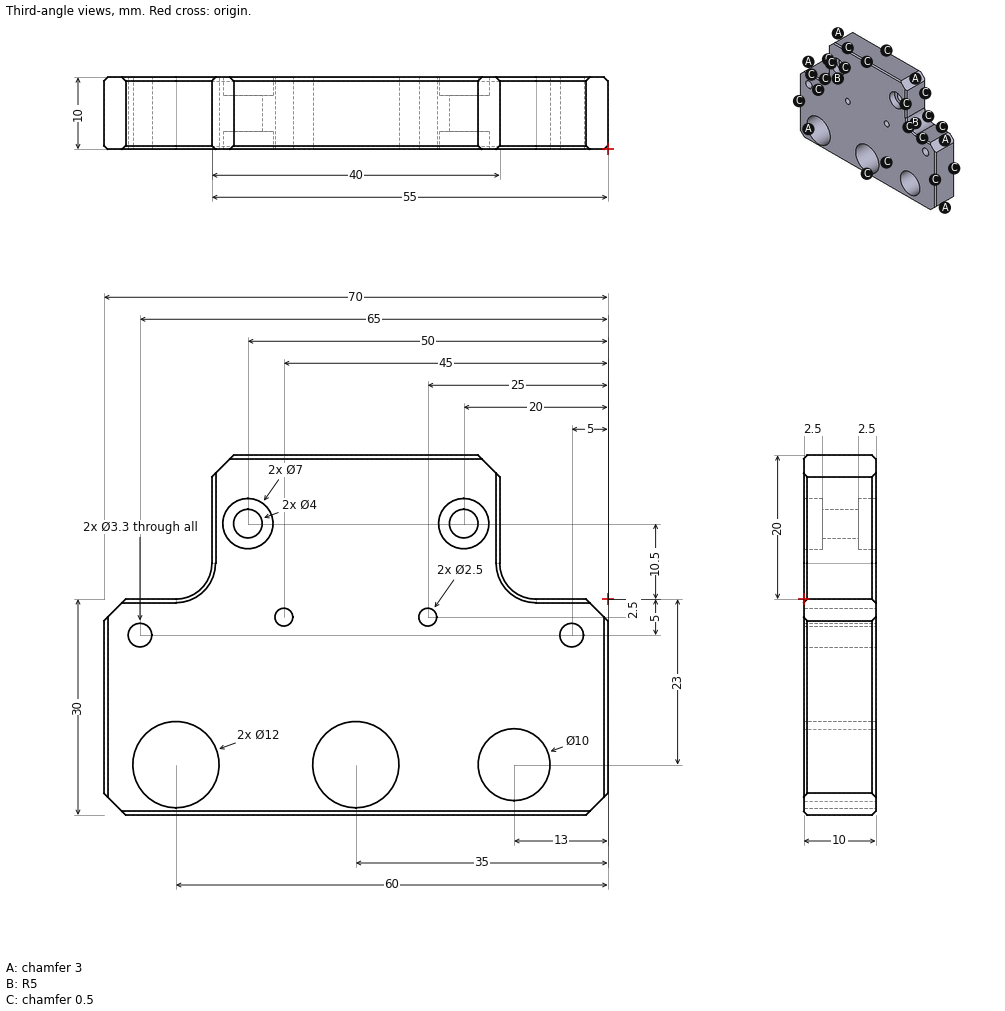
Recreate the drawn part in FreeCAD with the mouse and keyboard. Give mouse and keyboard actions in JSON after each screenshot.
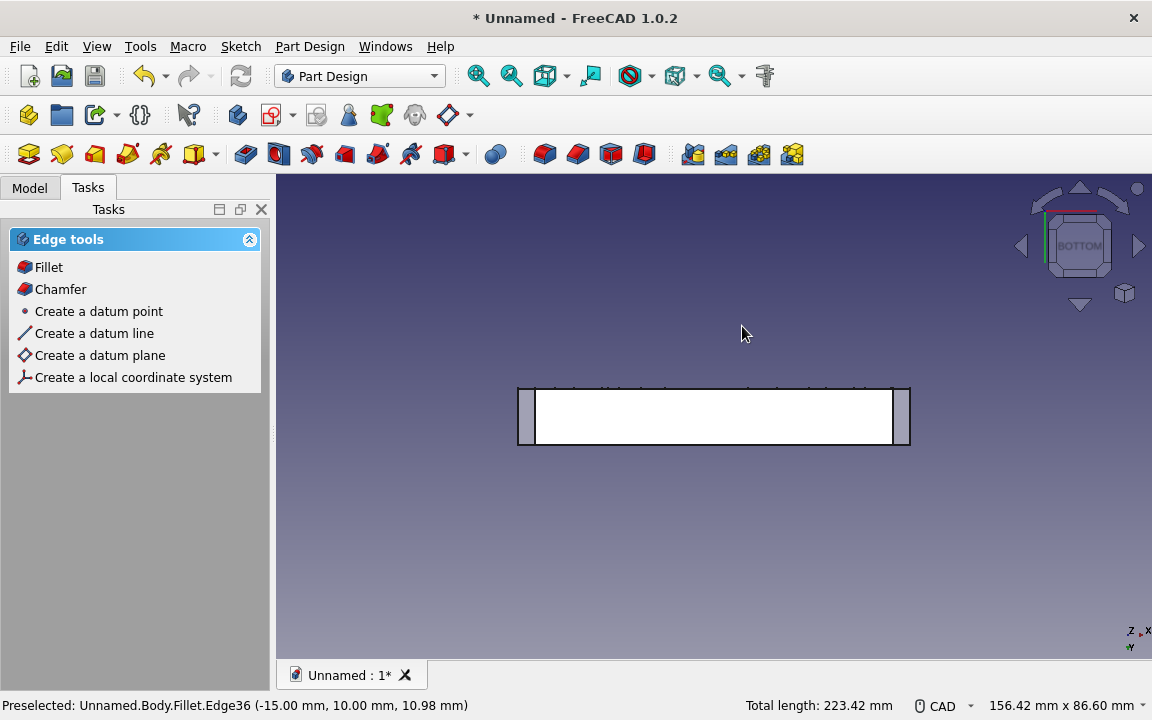
{"action": "left_click", "coordinate": [479, 76]}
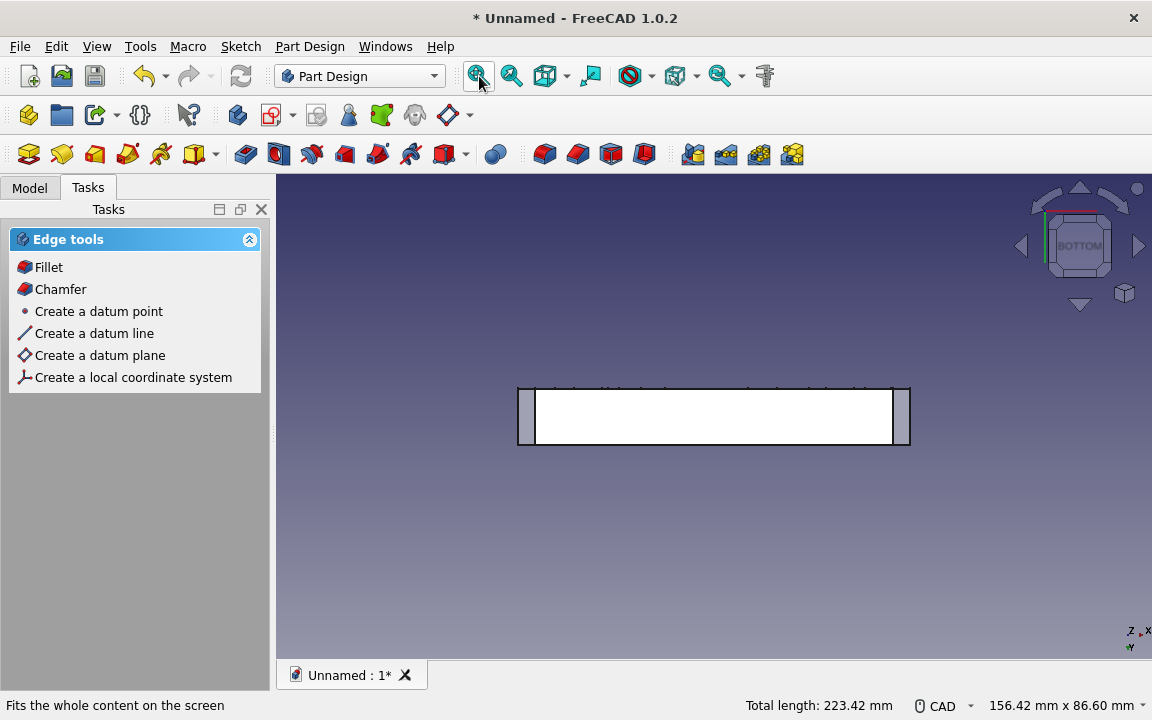
{"action": "left_click", "coordinate": [714, 387], "text": "ctrl"}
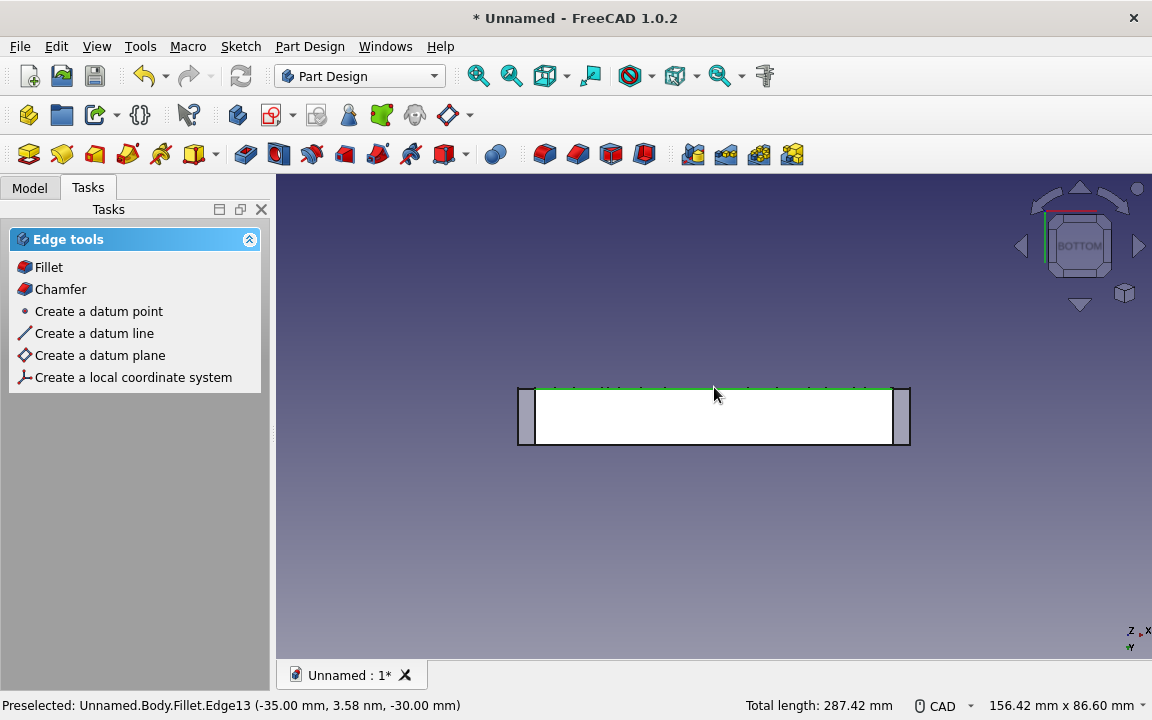
{"action": "key", "text": "4"}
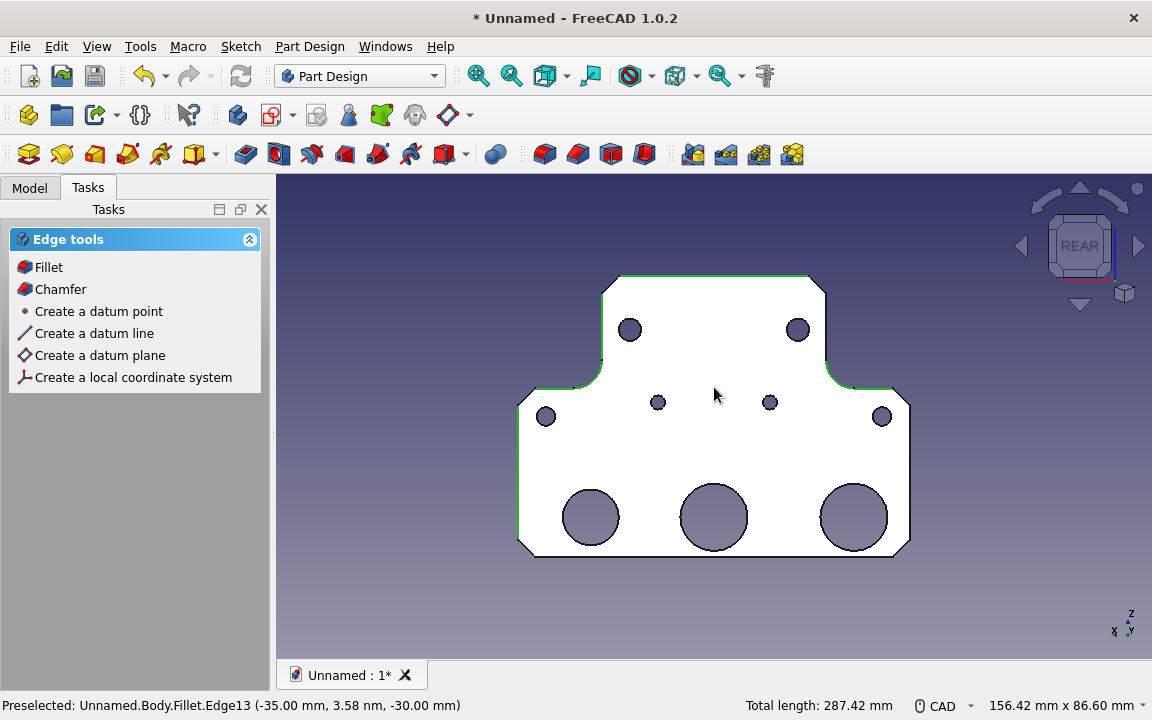
{"action": "left_click", "coordinate": [714, 556], "text": "ctrl"}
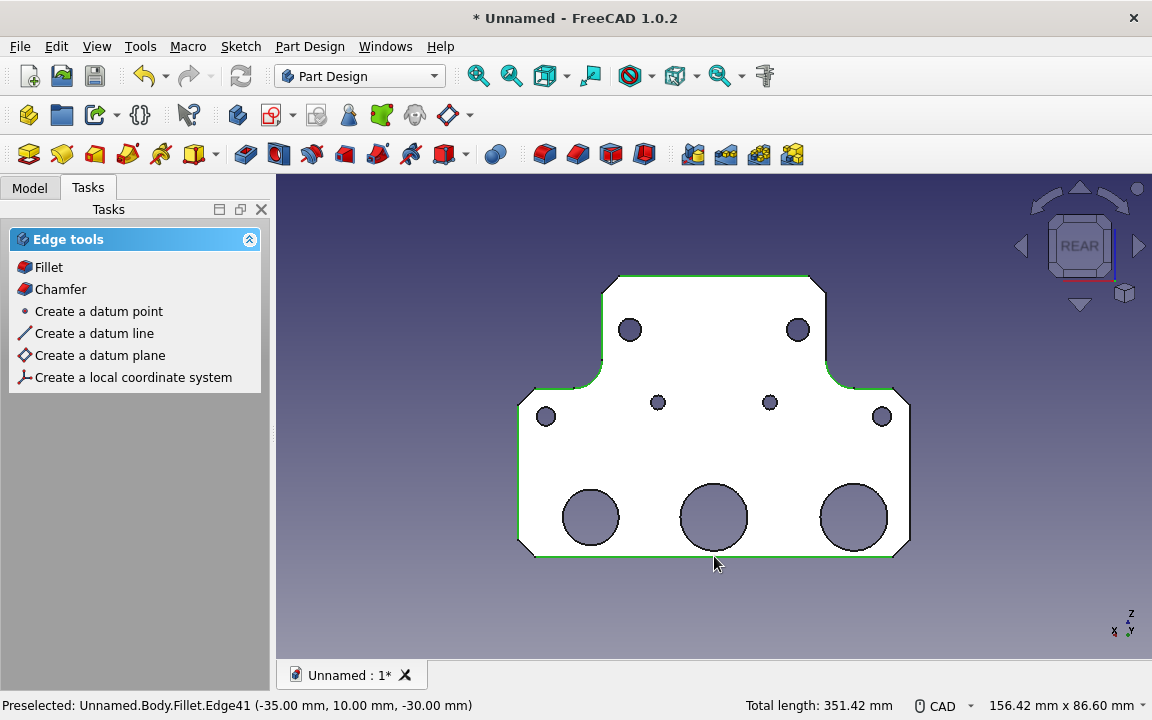
{"action": "left_click", "coordinate": [910, 472], "text": "ctrl"}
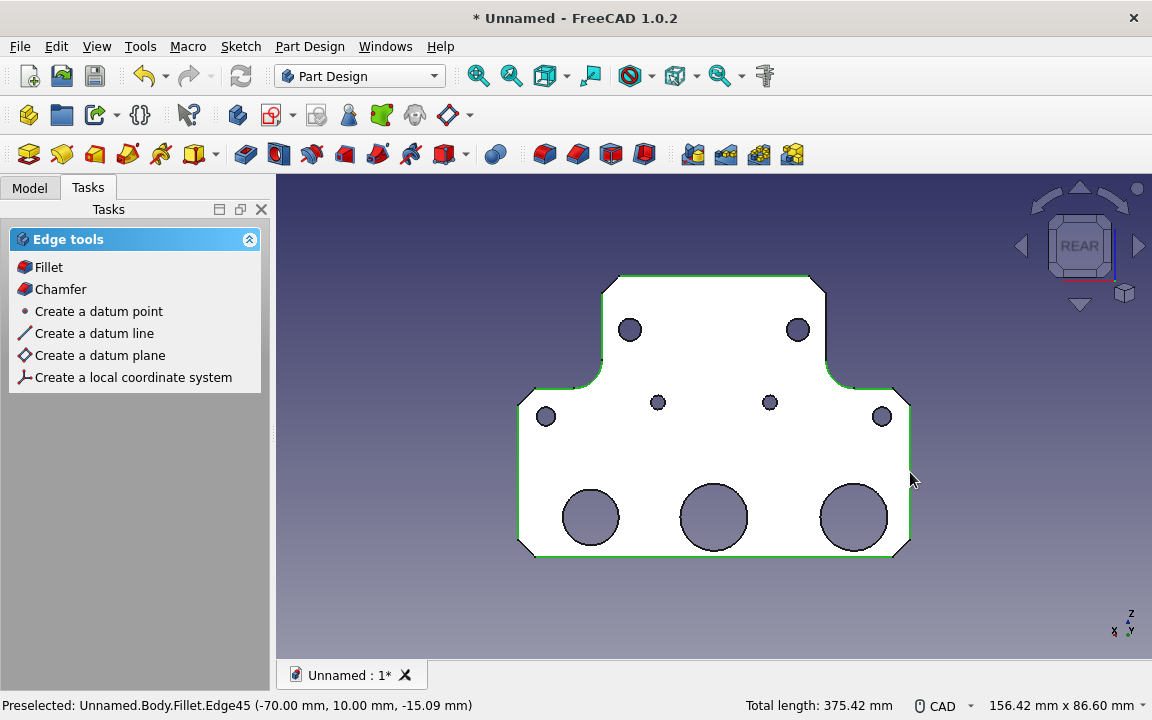
{"action": "left_click", "coordinate": [826, 326], "text": "ctrl"}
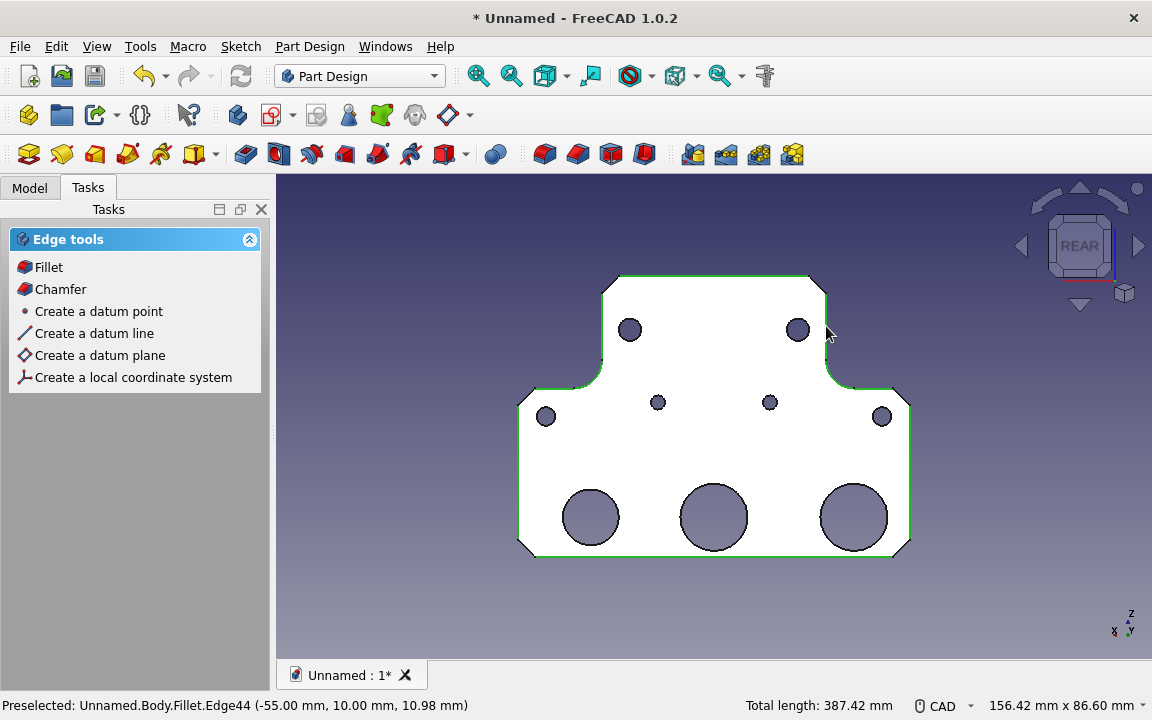
{"action": "key", "text": "6"}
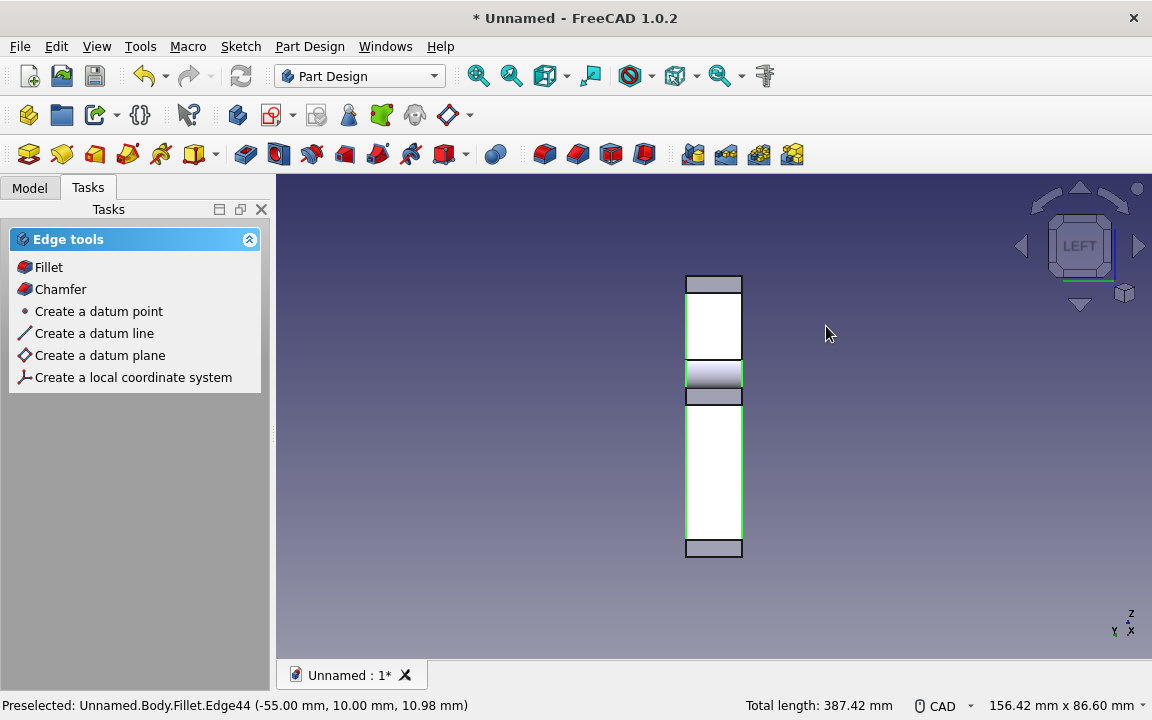
{"action": "left_click", "coordinate": [742, 326], "text": "ctrl"}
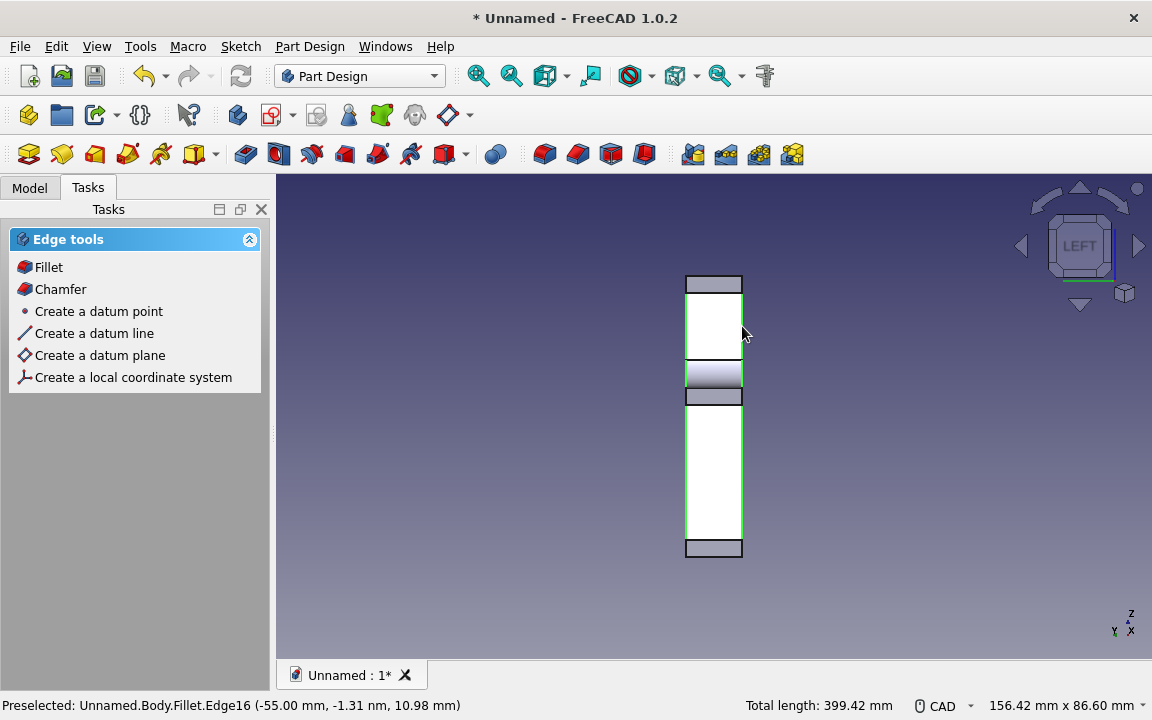
{"action": "left_click", "coordinate": [578, 154]}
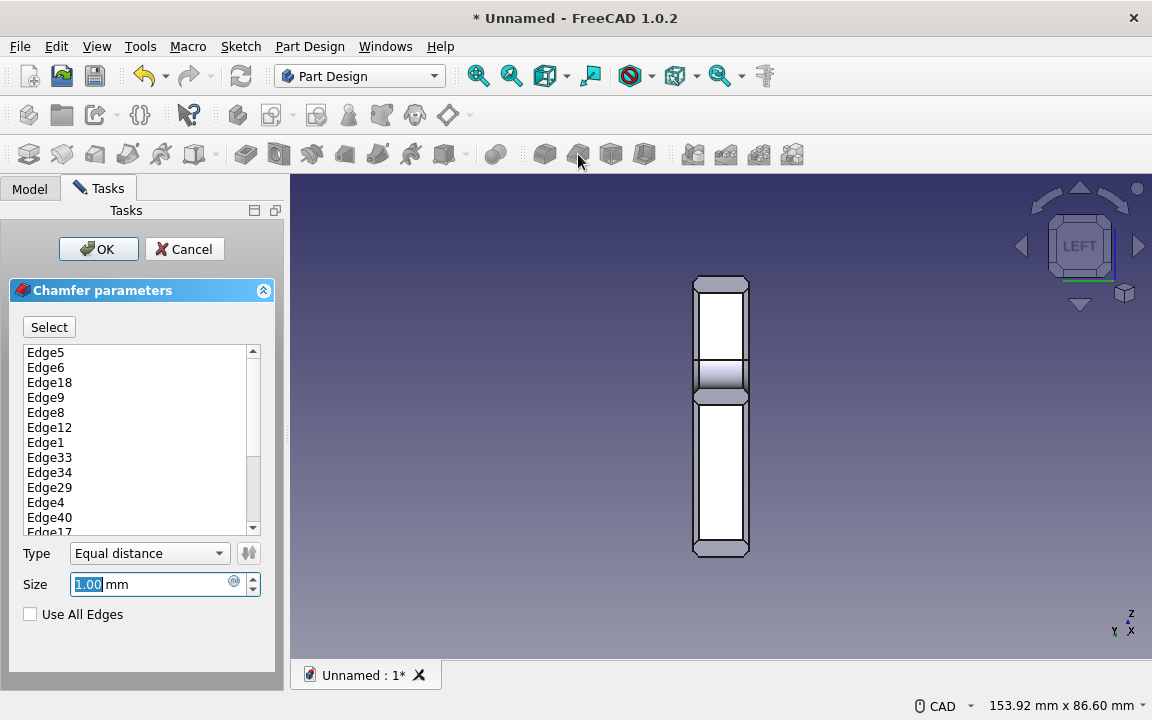
{"action": "type", "text": "0.5"}
{"action": "key", "text": "Tab"}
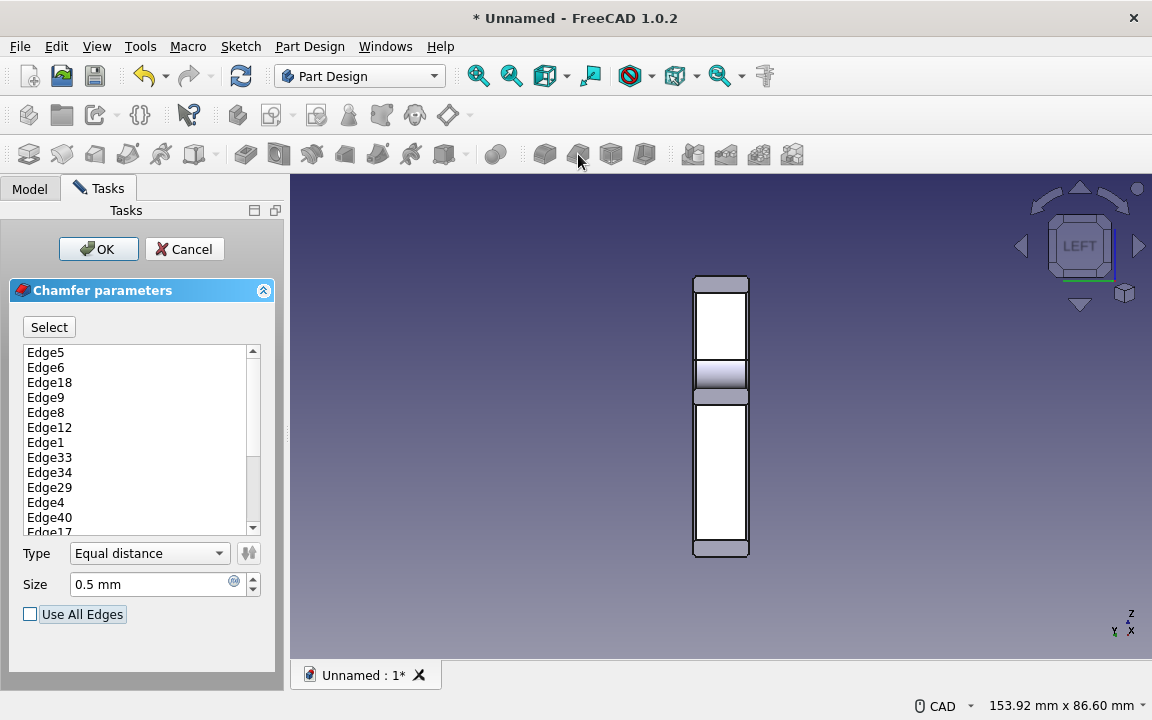
{"action": "left_click", "coordinate": [99, 249]}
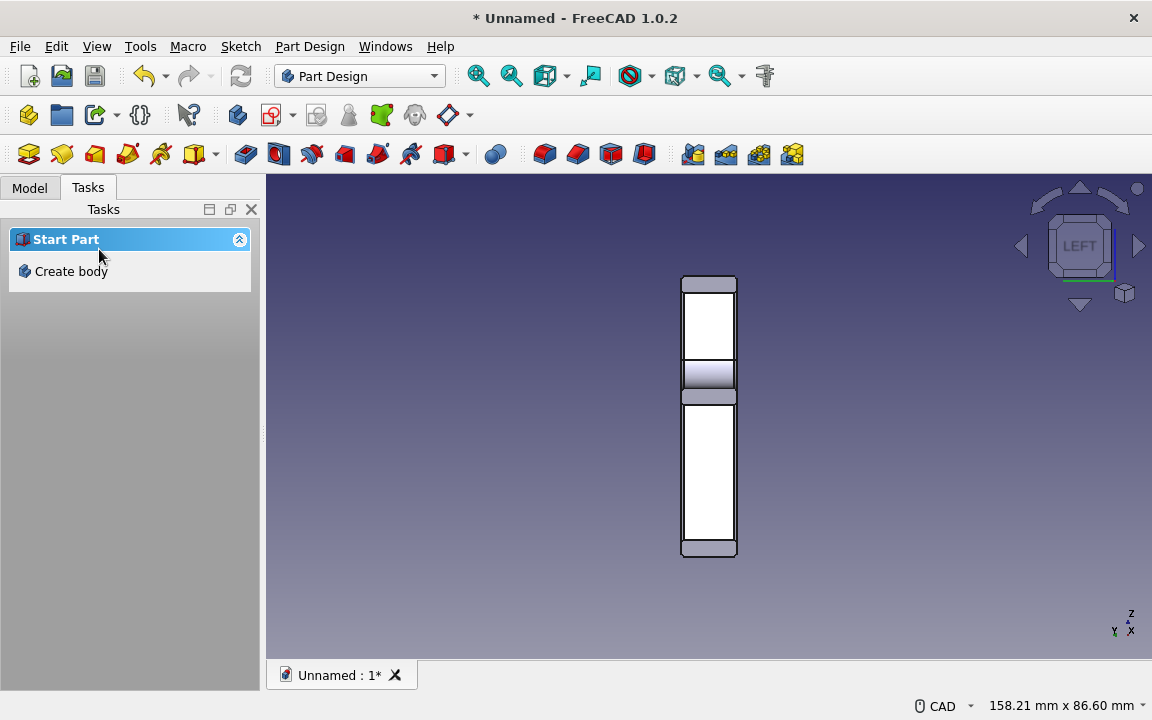
{"action": "key", "text": "4"}